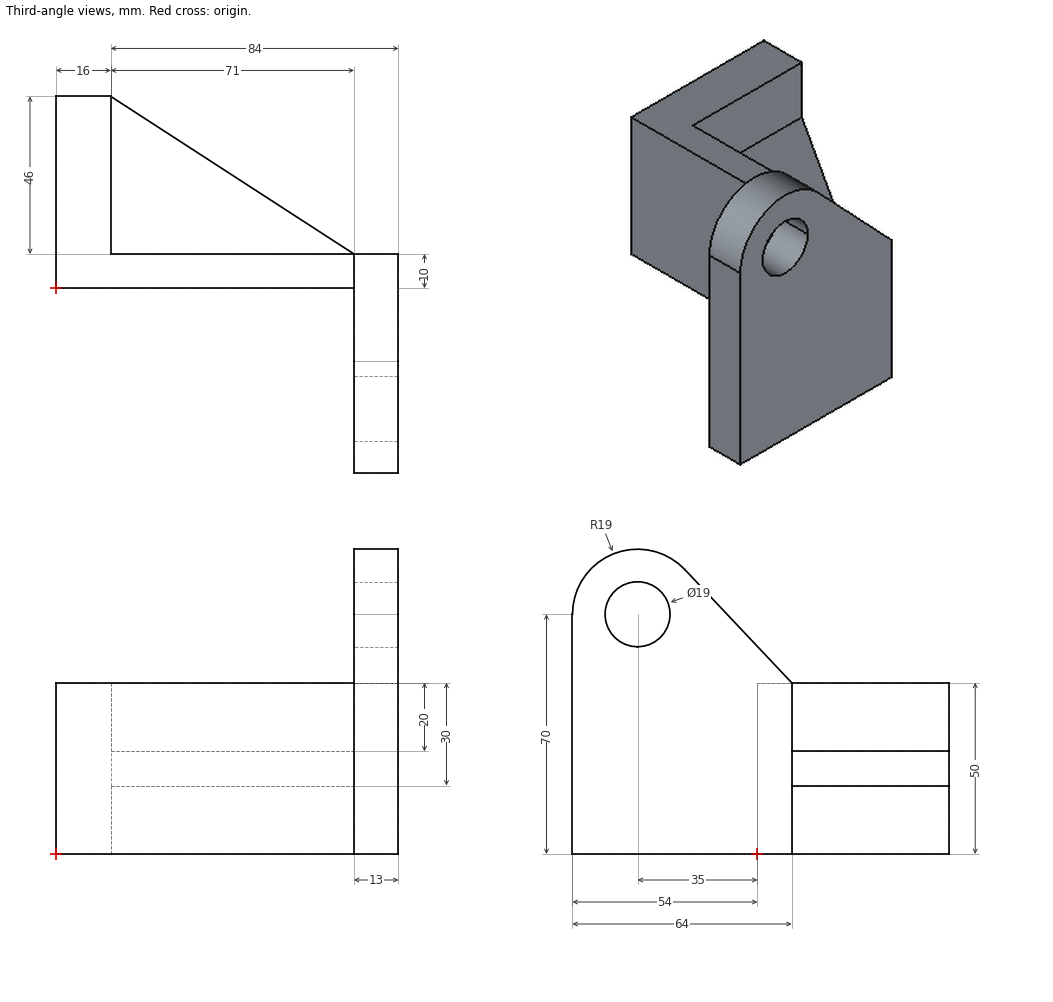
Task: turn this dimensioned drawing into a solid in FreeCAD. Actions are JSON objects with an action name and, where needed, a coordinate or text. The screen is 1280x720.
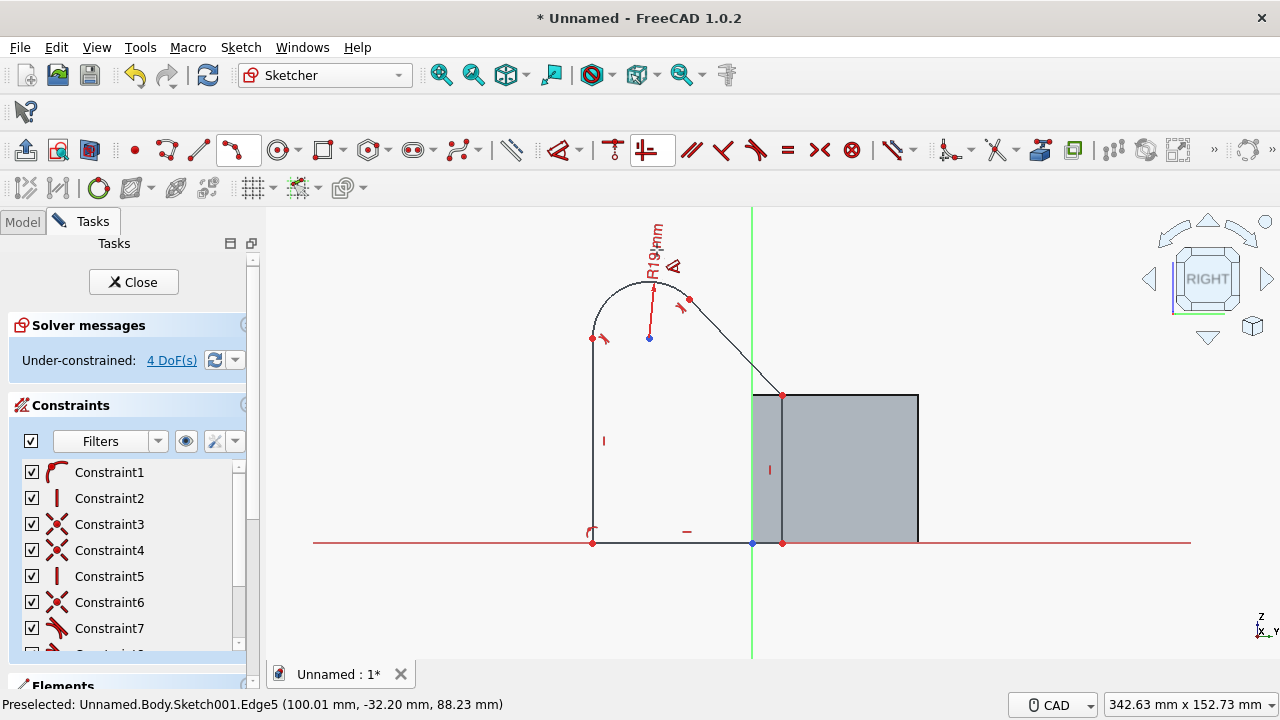
{"action": "left_click", "coordinate": [593, 400]}
{"action": "left_click", "coordinate": [559, 441]}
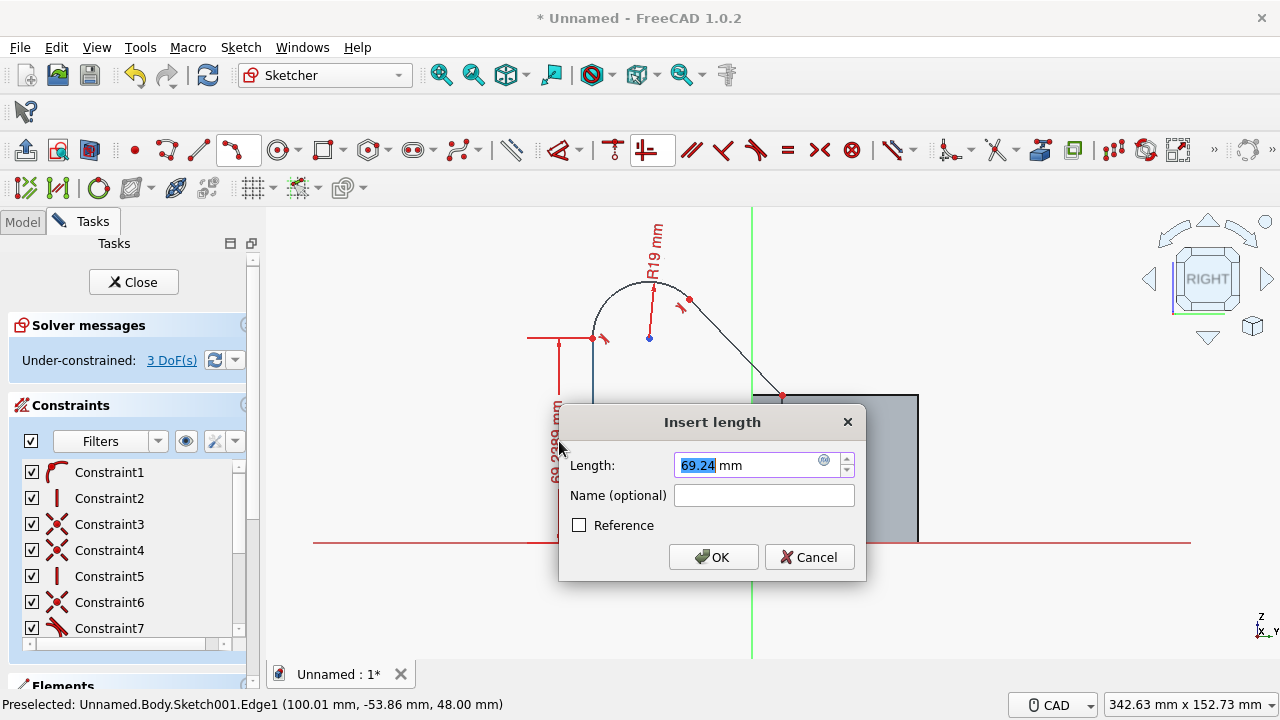
{"action": "type", "text": "70"}
{"action": "key", "text": "Return"}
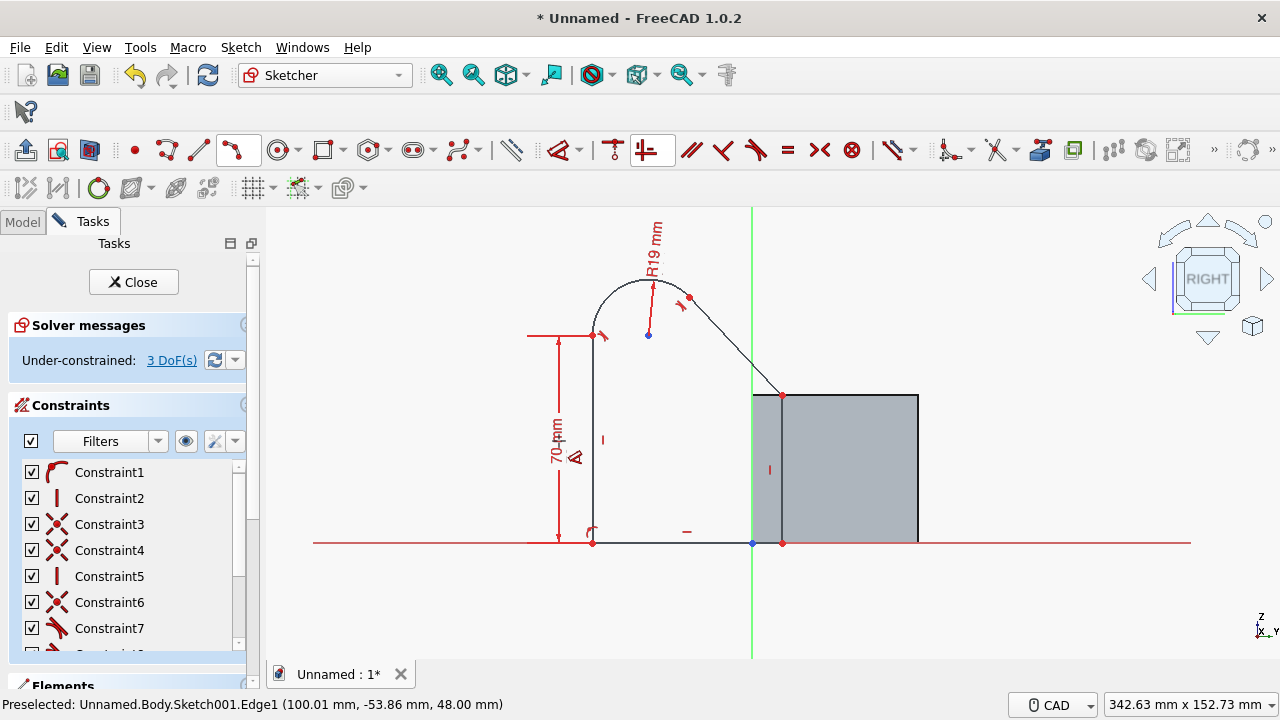
{"action": "left_click", "coordinate": [649, 543]}
{"action": "left_click", "coordinate": [687, 577]}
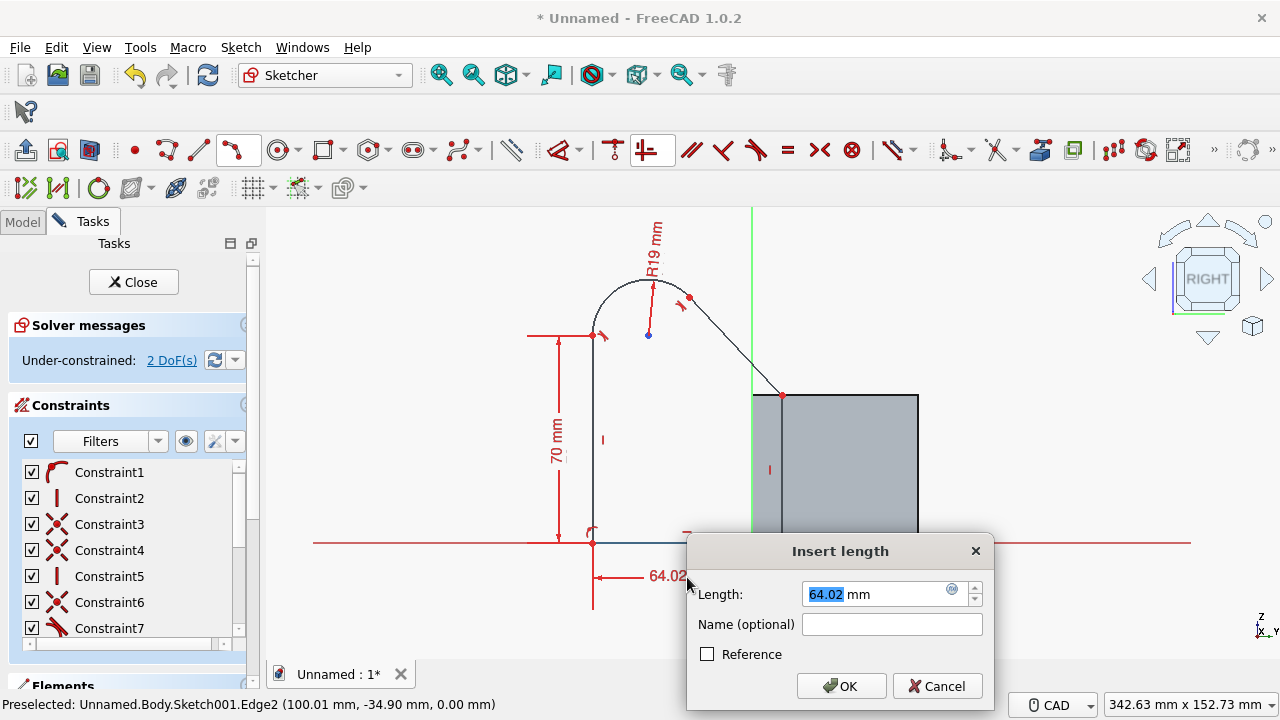
{"action": "type", "text": "64"}
{"action": "key", "text": "Return"}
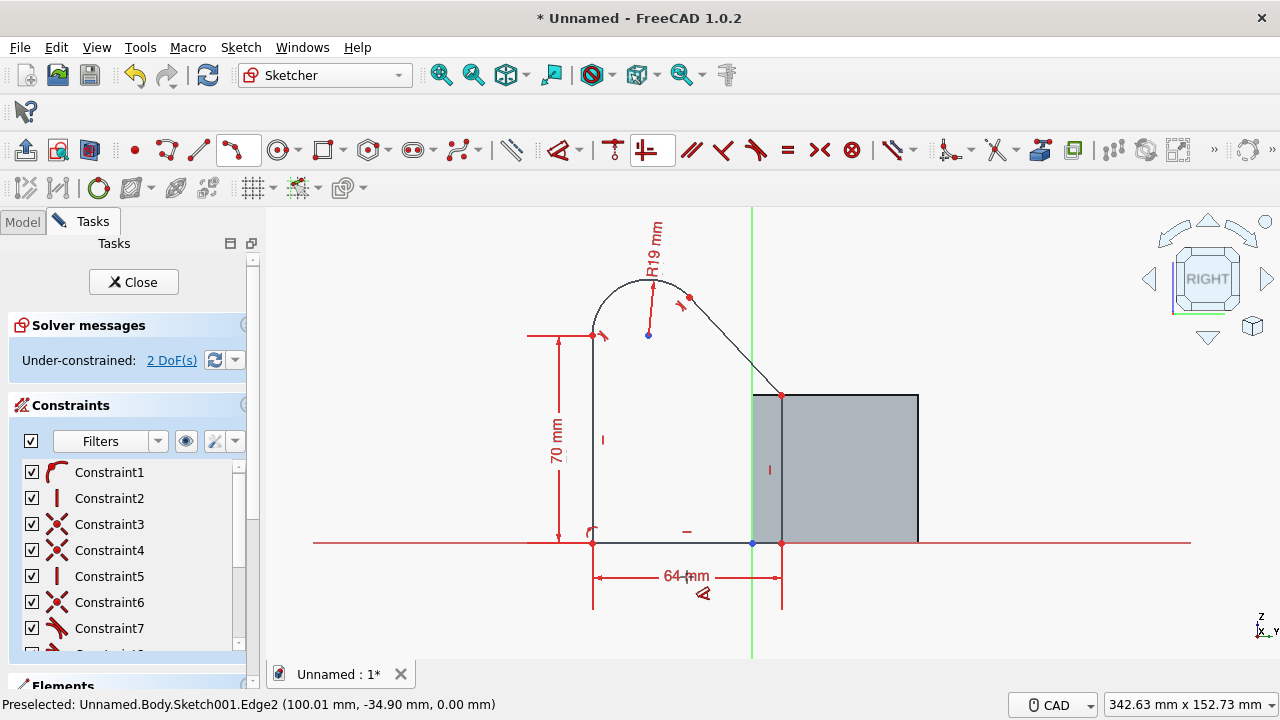
{"action": "left_click", "coordinate": [782, 499]}
{"action": "left_click", "coordinate": [816, 470]}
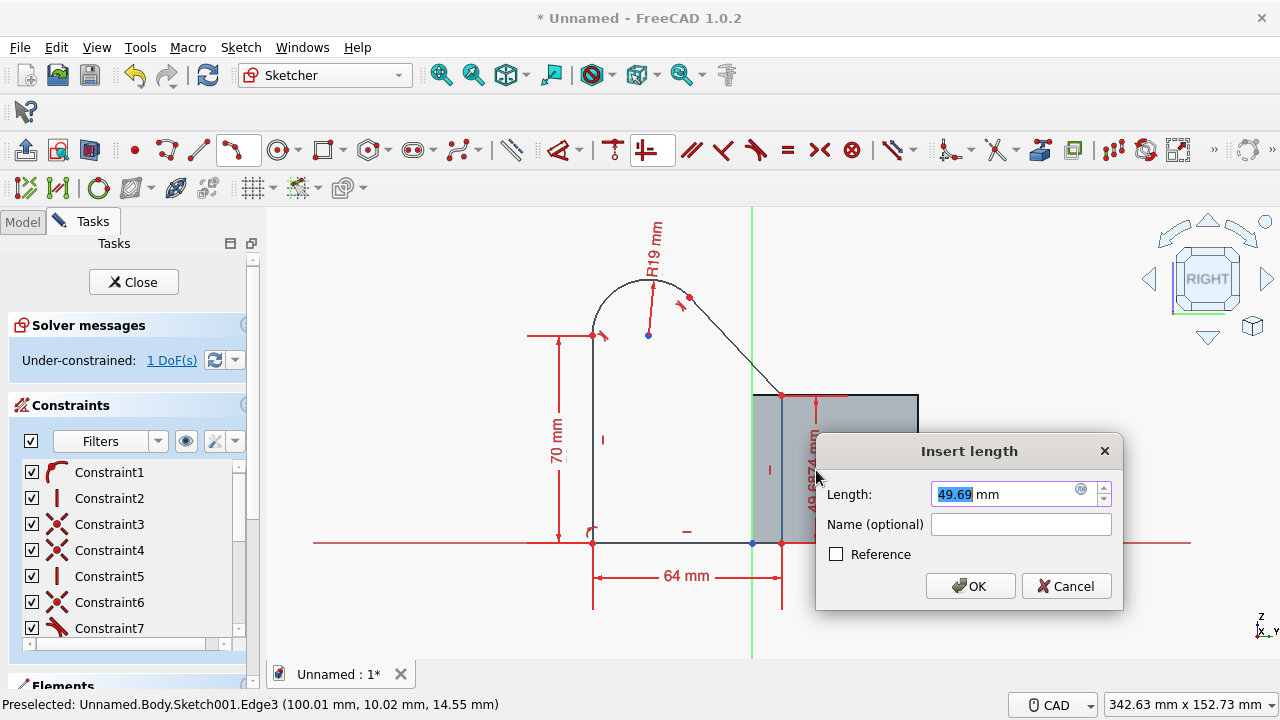
{"action": "type", "text": "50"}
{"action": "key", "text": "Return"}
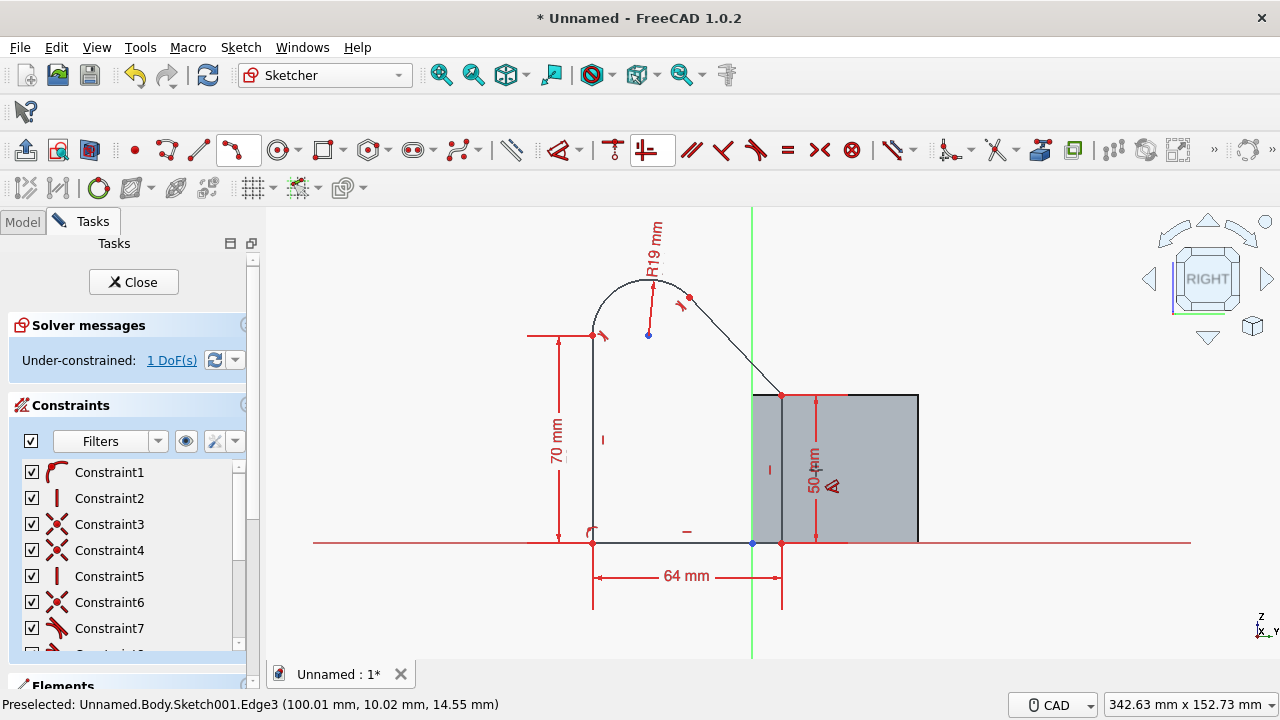
{"action": "left_click", "coordinate": [593, 336]}
{"action": "left_click", "coordinate": [616, 577]}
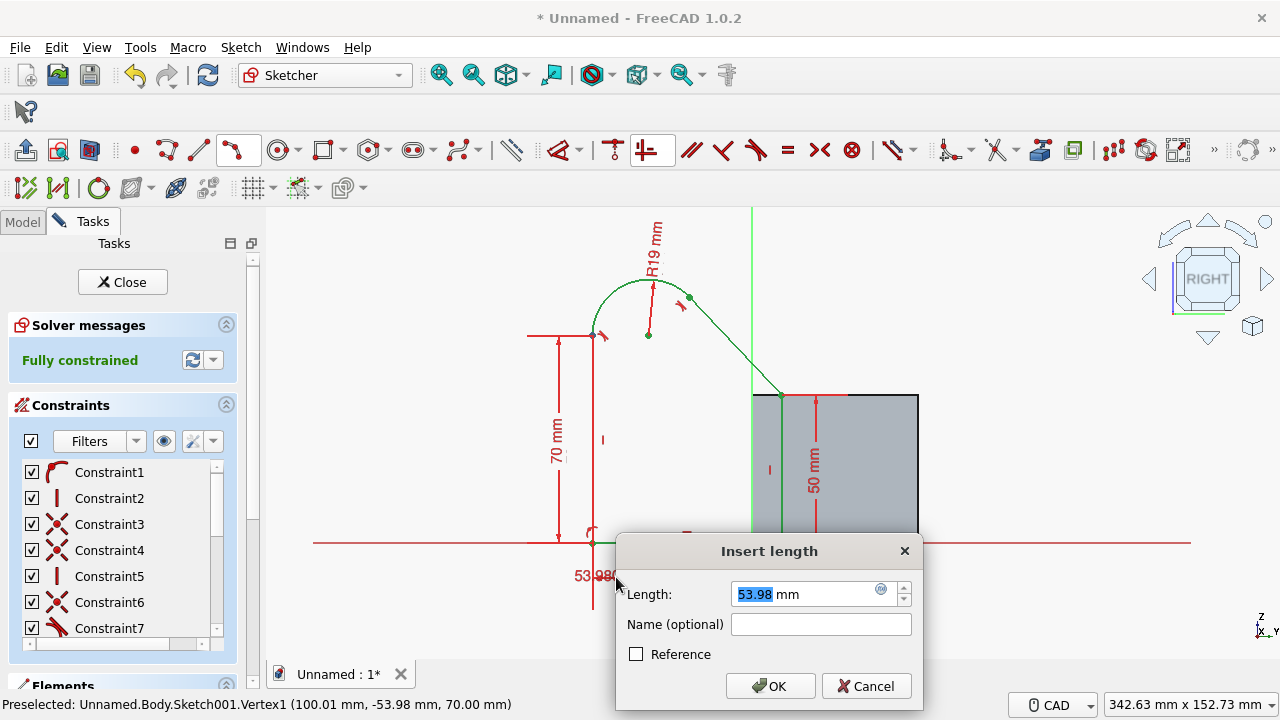
{"action": "type", "text": "54"}
{"action": "key", "text": "Return"}
{"action": "key", "text": "Escape"}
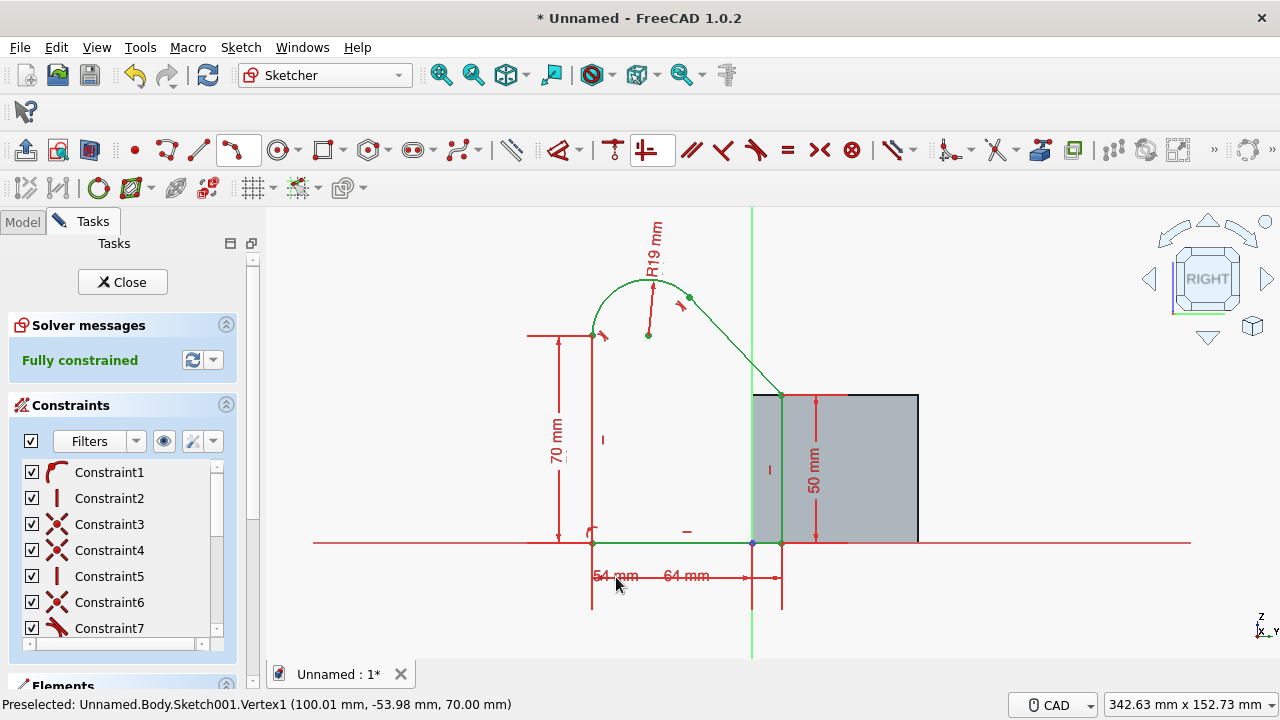
{"action": "left_click", "coordinate": [123, 282]}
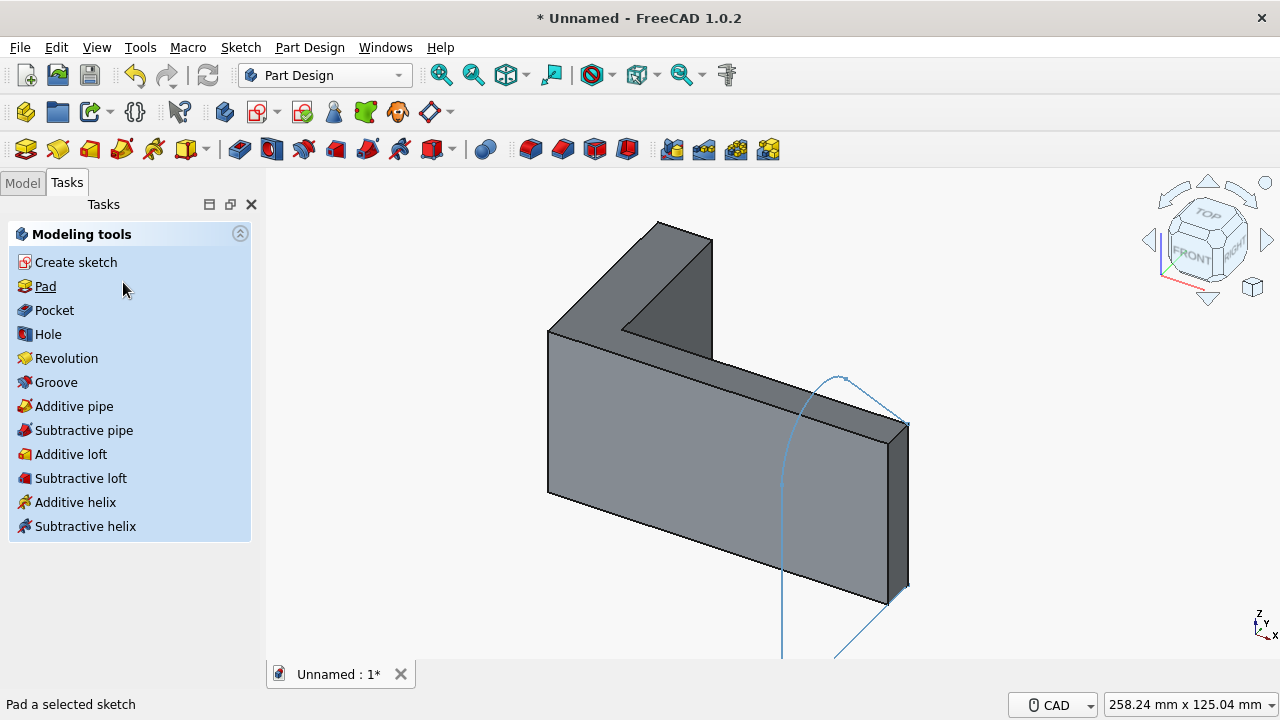
{"action": "left_click", "coordinate": [26, 150]}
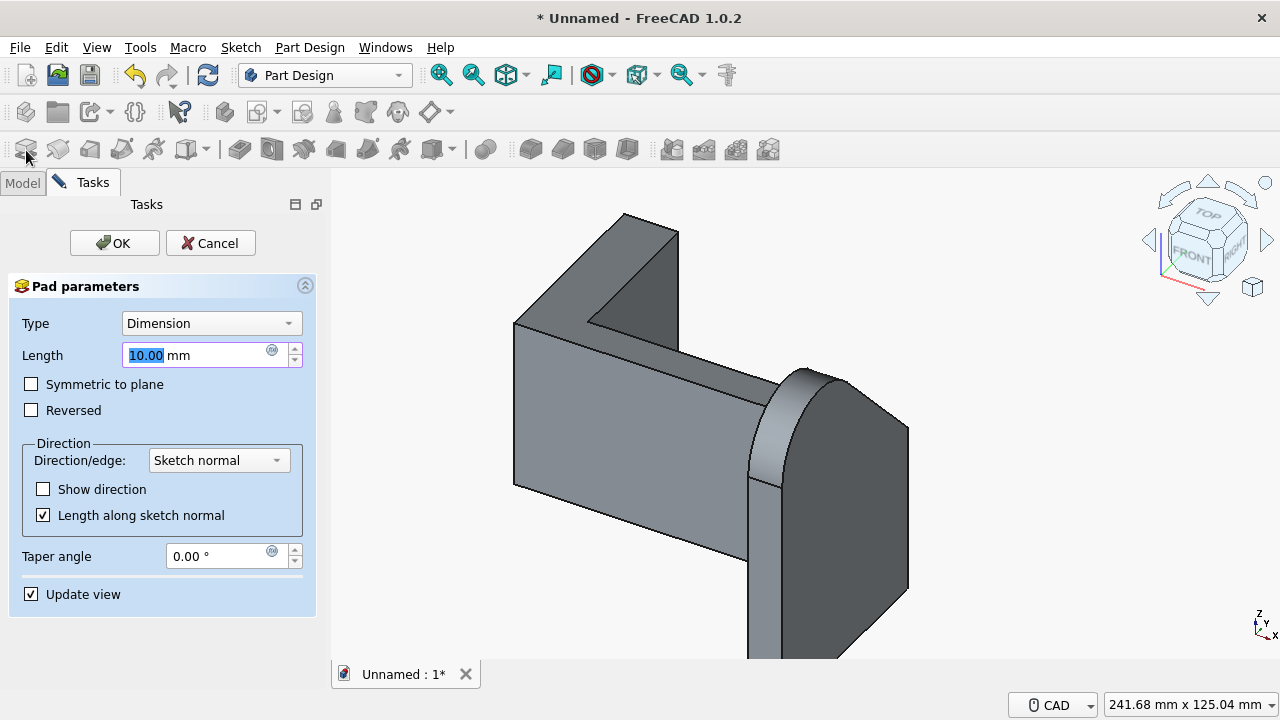
{"action": "type", "text": "13"}
{"action": "key", "text": "Tab"}